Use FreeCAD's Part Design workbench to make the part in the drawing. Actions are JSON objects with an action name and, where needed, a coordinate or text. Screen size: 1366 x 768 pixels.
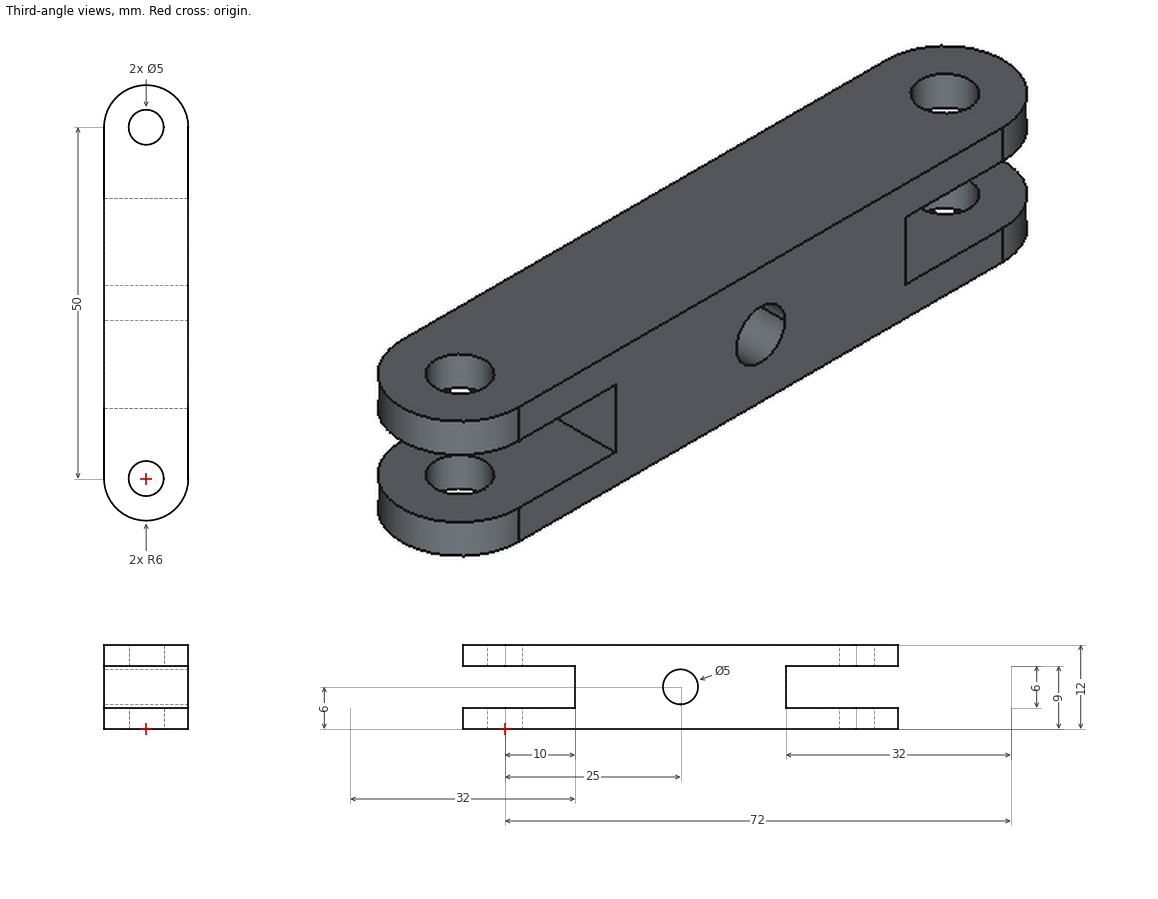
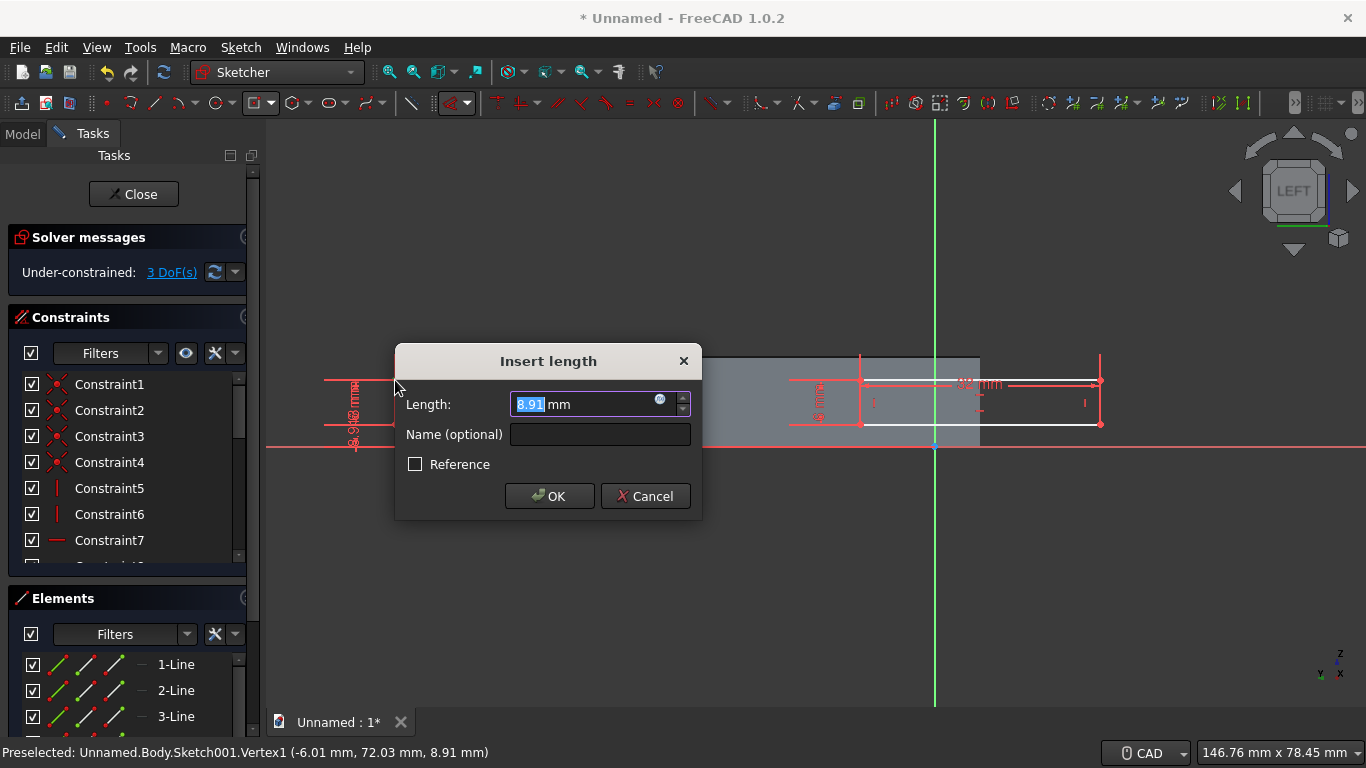
{"action": "type", "text": "9"}
{"action": "key", "text": "Return"}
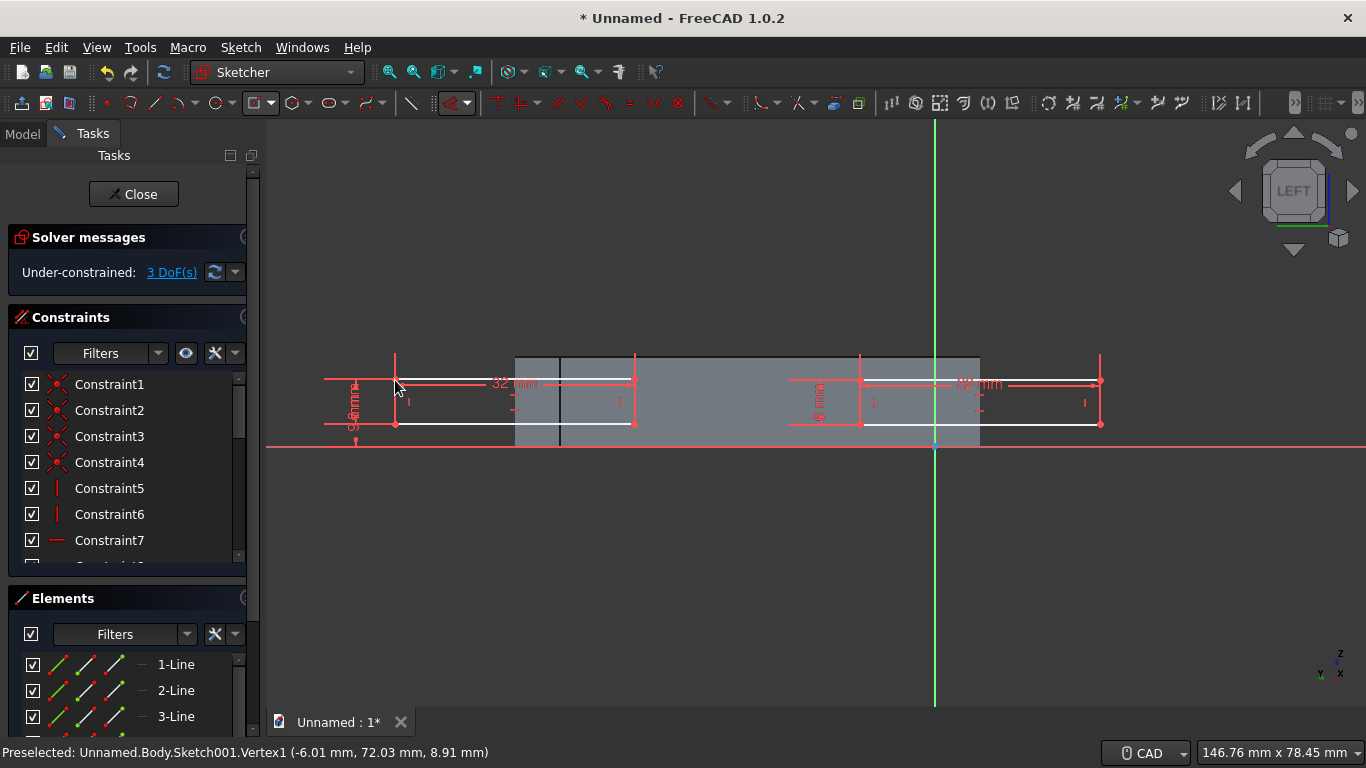
{"action": "left_click", "coordinate": [860, 380]}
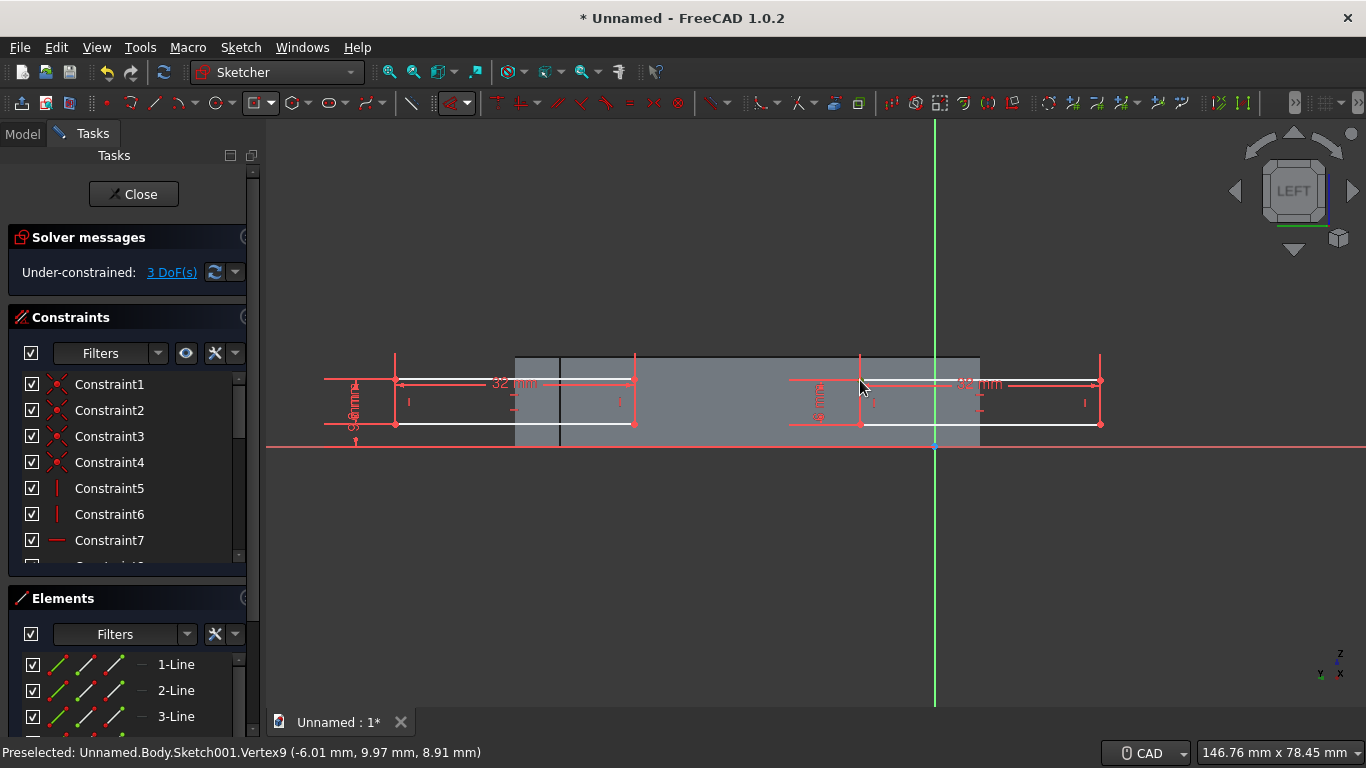
{"action": "key", "text": "i"}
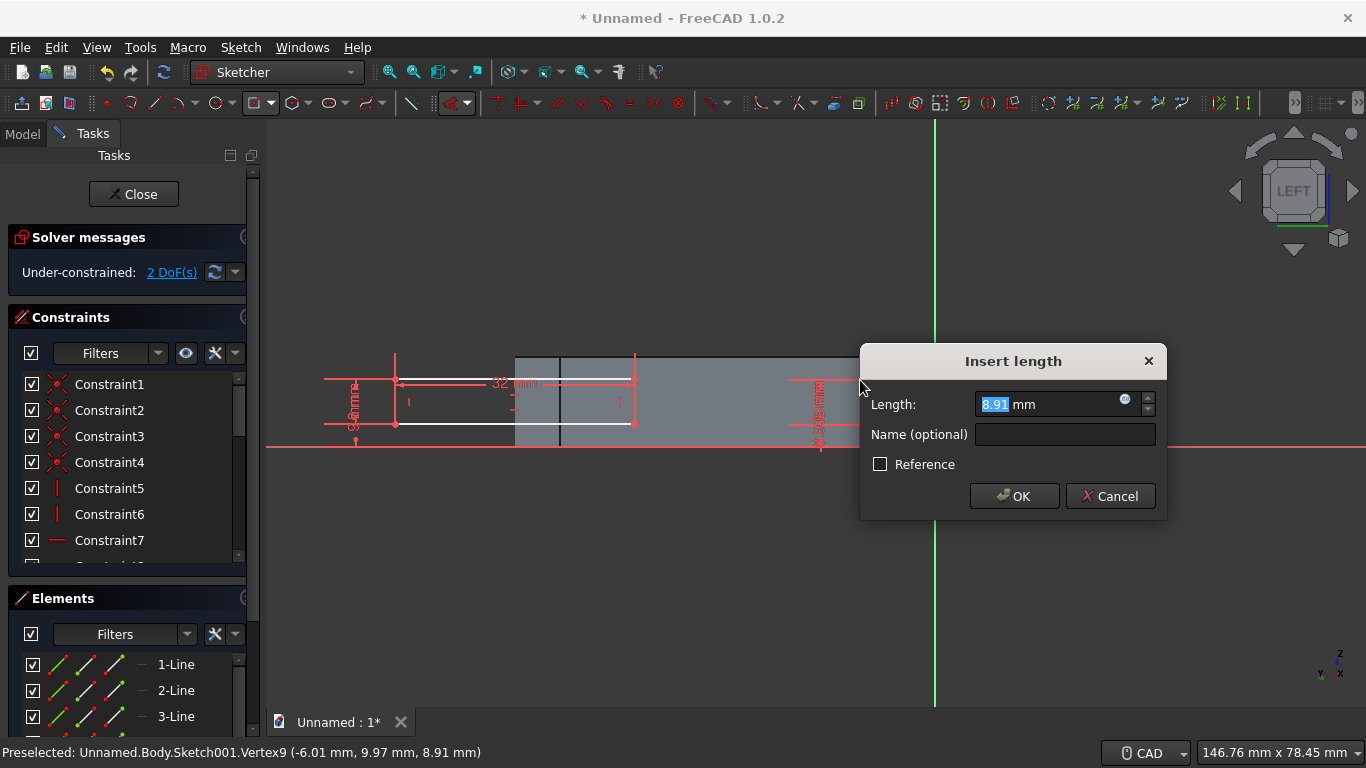
{"action": "type", "text": "9"}
{"action": "key", "text": "Return"}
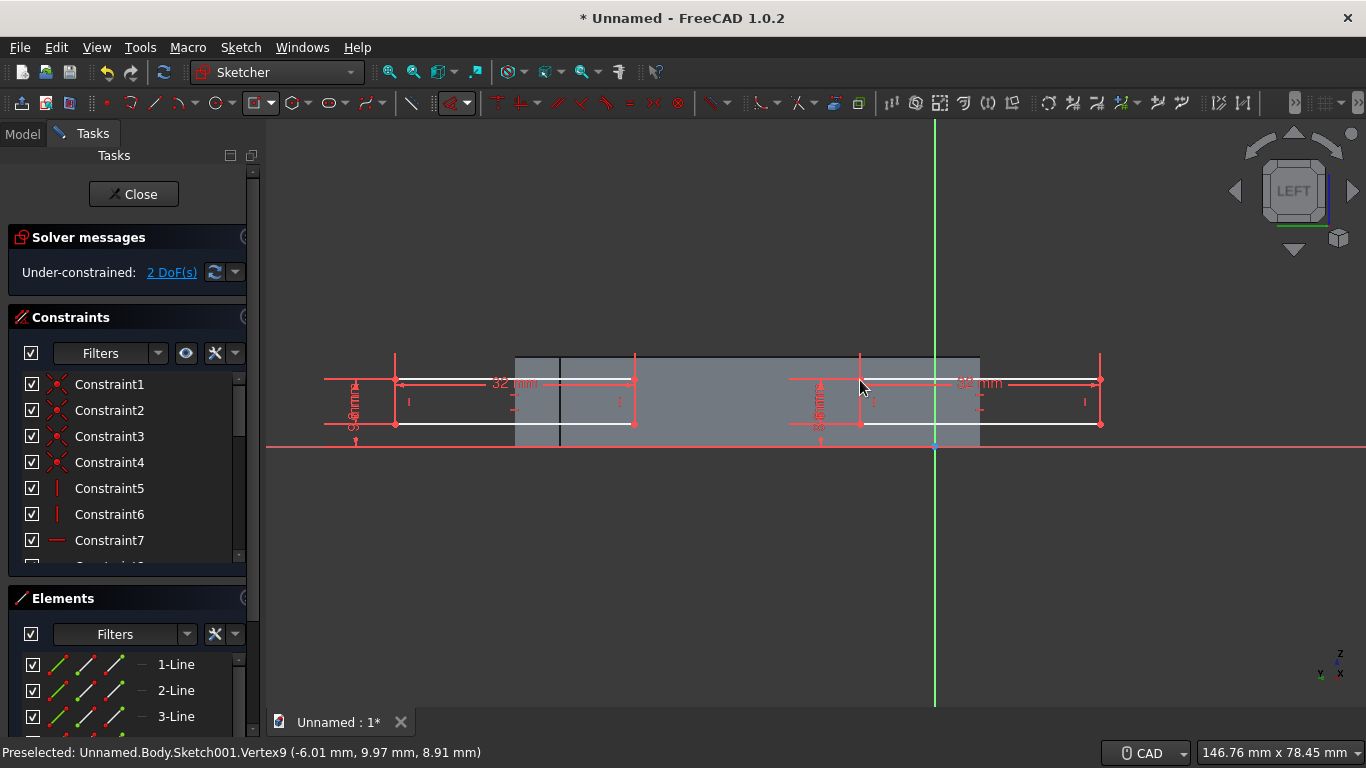
{"action": "left_click", "coordinate": [395, 379]}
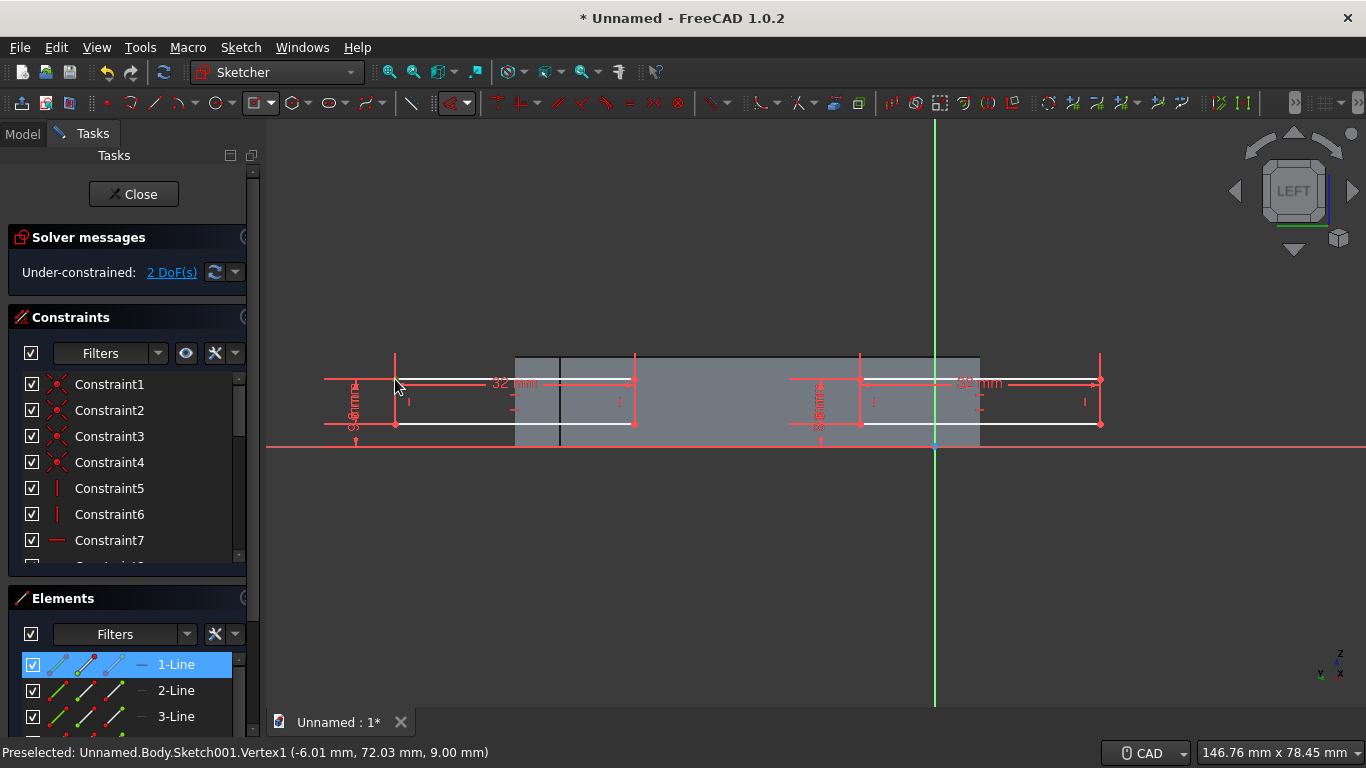
{"action": "key", "text": "l"}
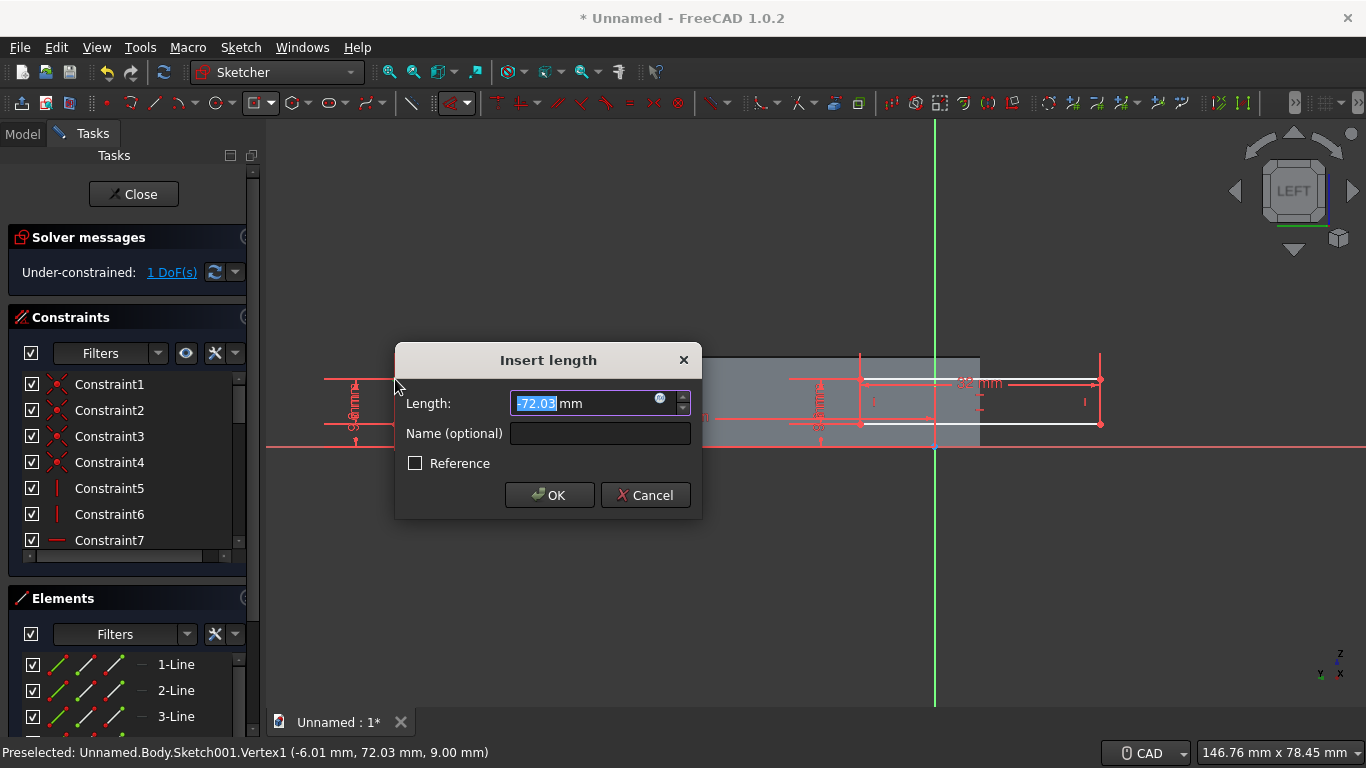
{"action": "type", "text": "-72"}
{"action": "key", "text": "Return"}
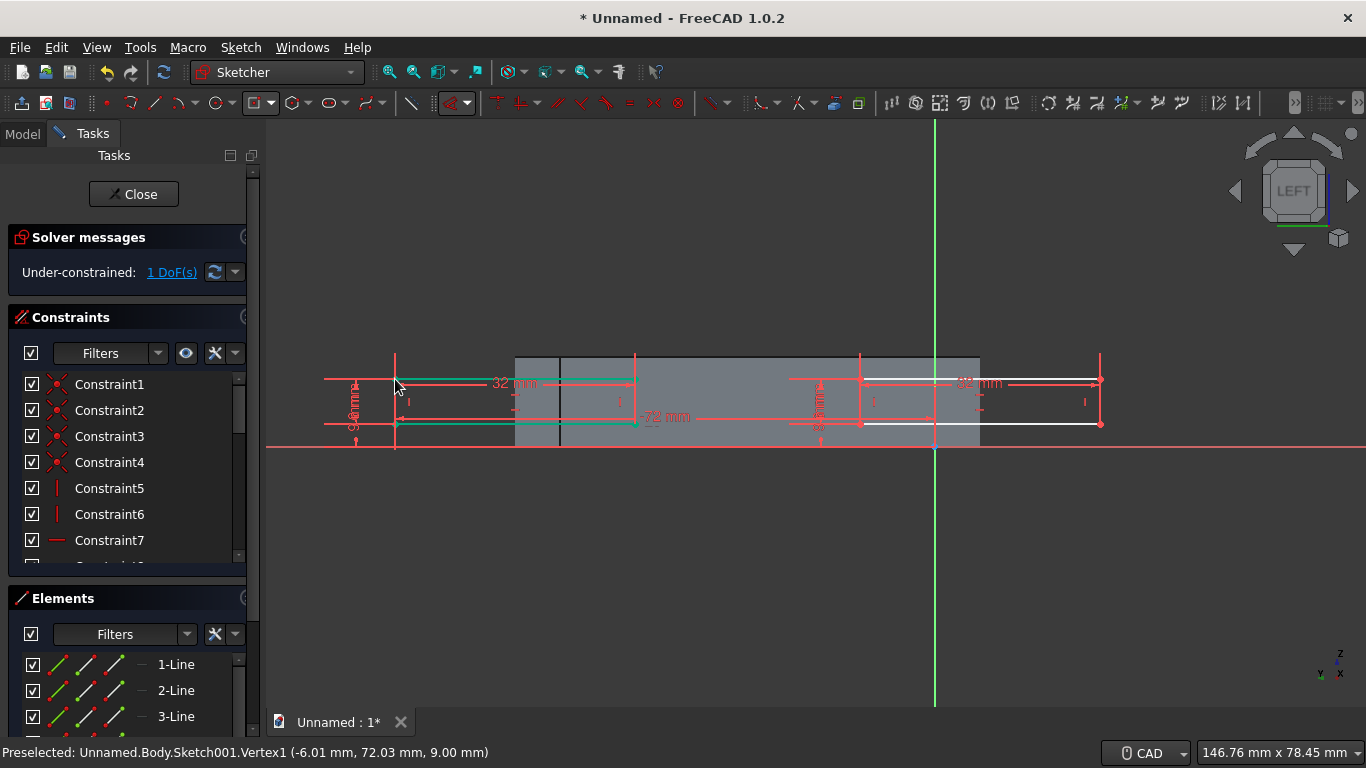
{"action": "left_click", "coordinate": [860, 379]}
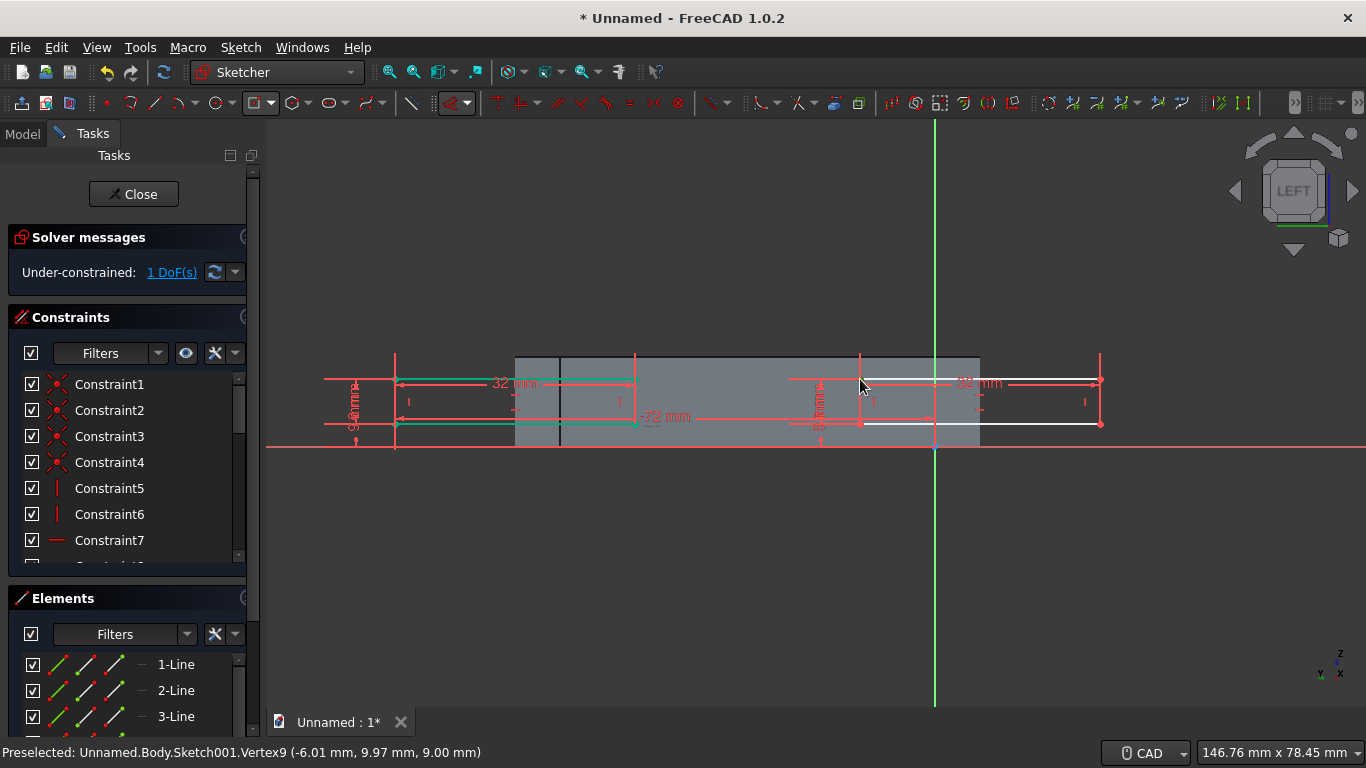
{"action": "key", "text": "l"}